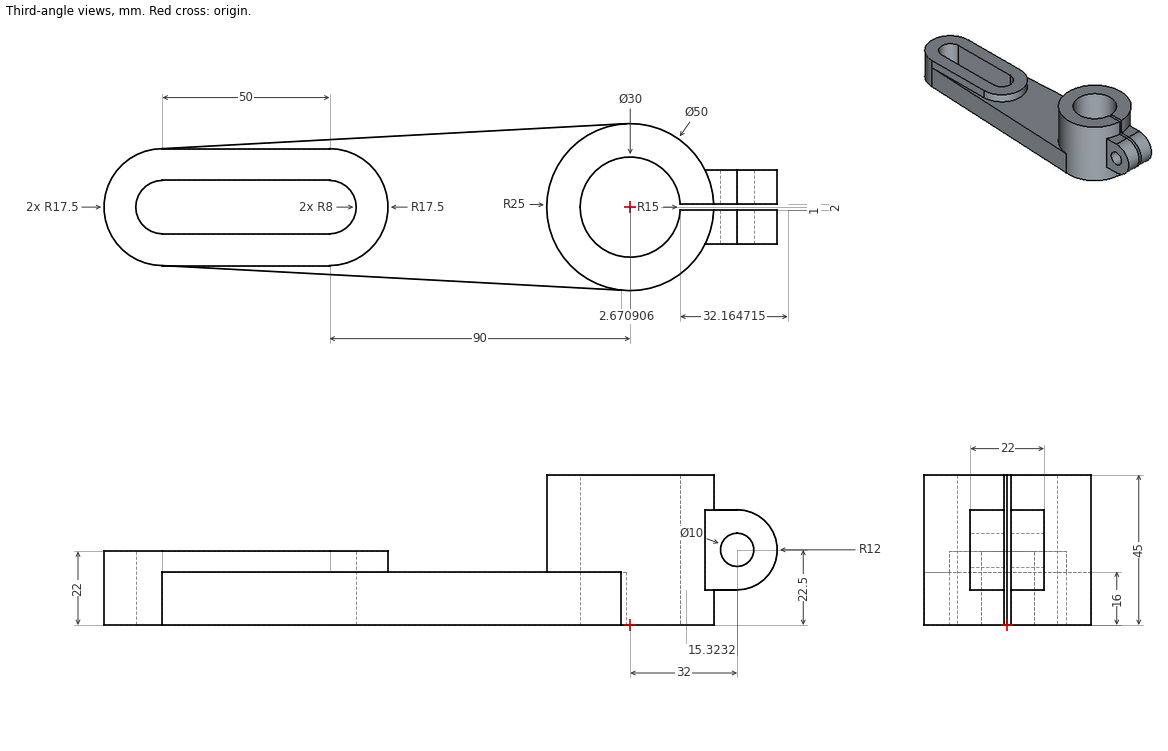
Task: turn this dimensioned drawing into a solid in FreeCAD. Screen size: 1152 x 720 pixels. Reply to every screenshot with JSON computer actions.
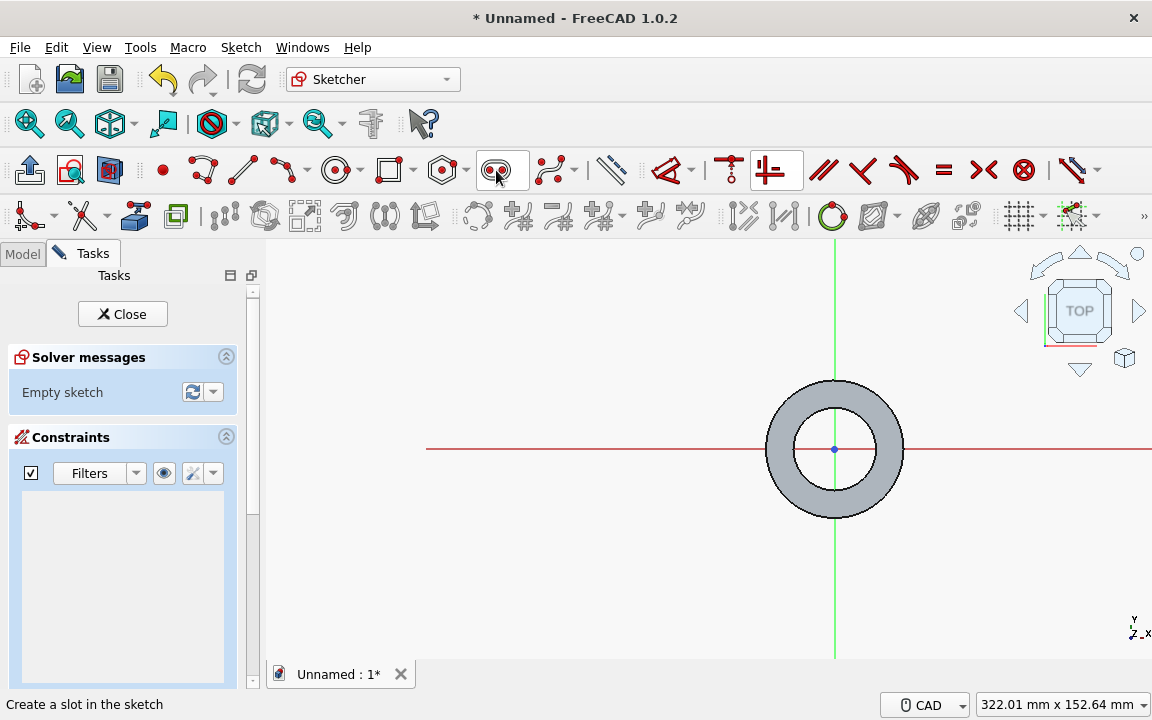
{"action": "left_click", "coordinate": [450, 449]}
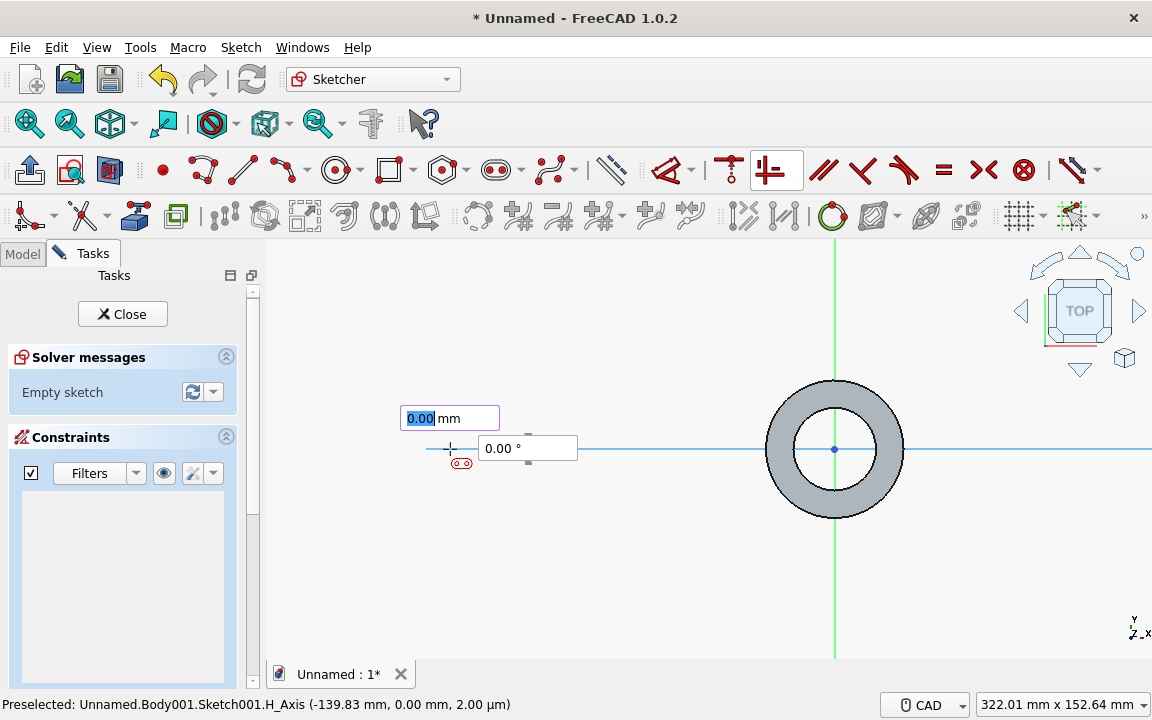
{"action": "left_click", "coordinate": [587, 440]}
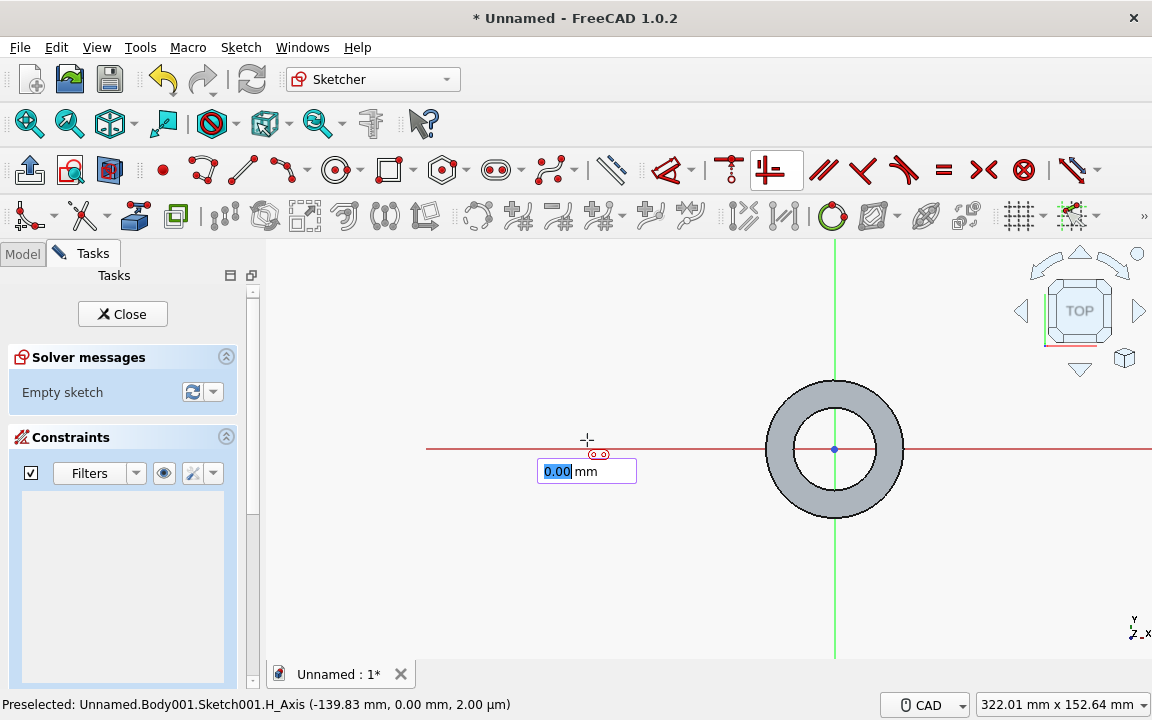
{"action": "left_click", "coordinate": [518, 401]}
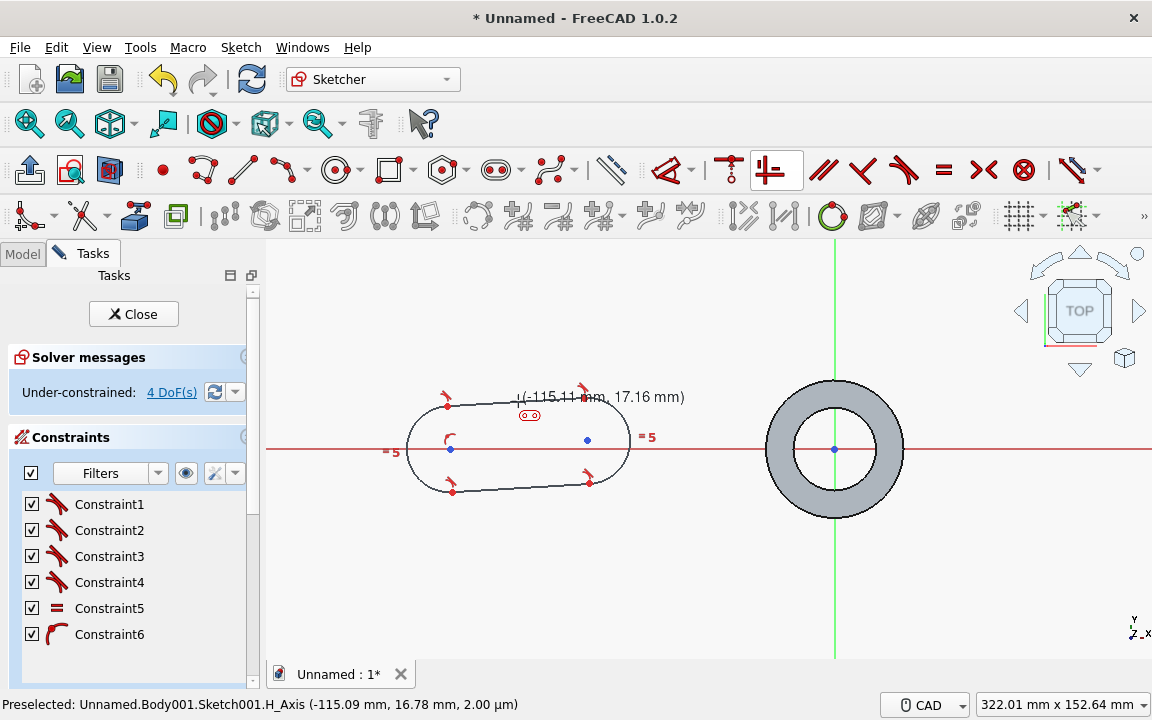
{"action": "left_click", "coordinate": [450, 449]}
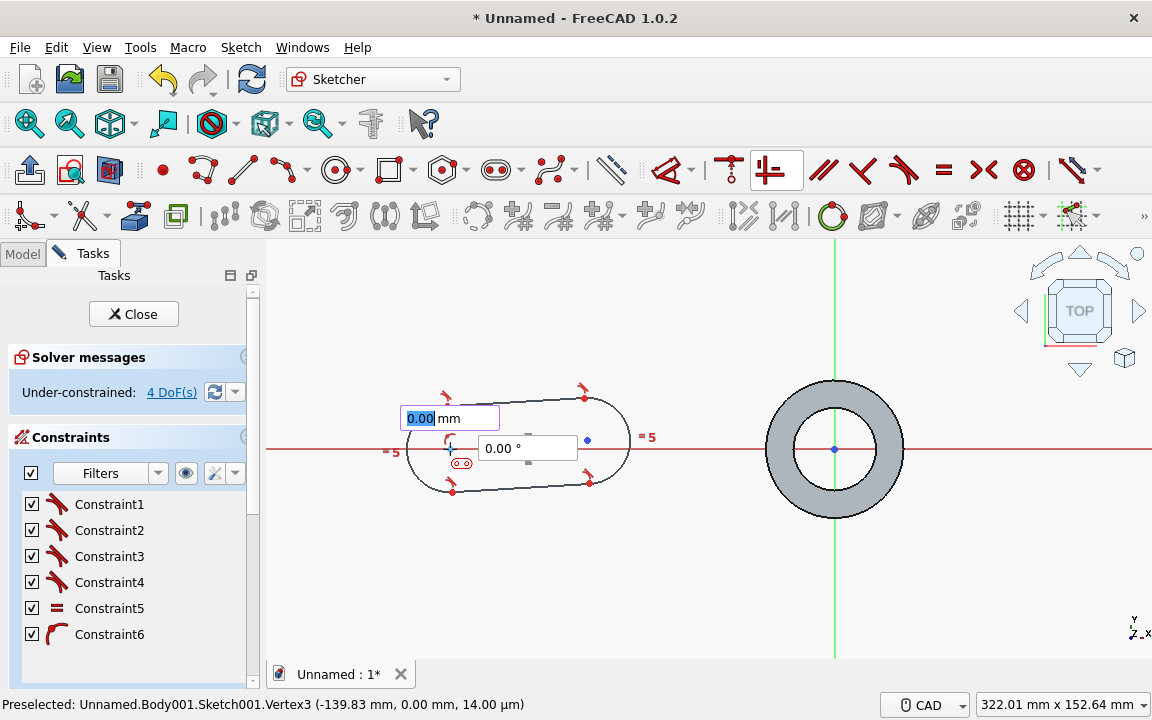
{"action": "left_click", "coordinate": [587, 441]}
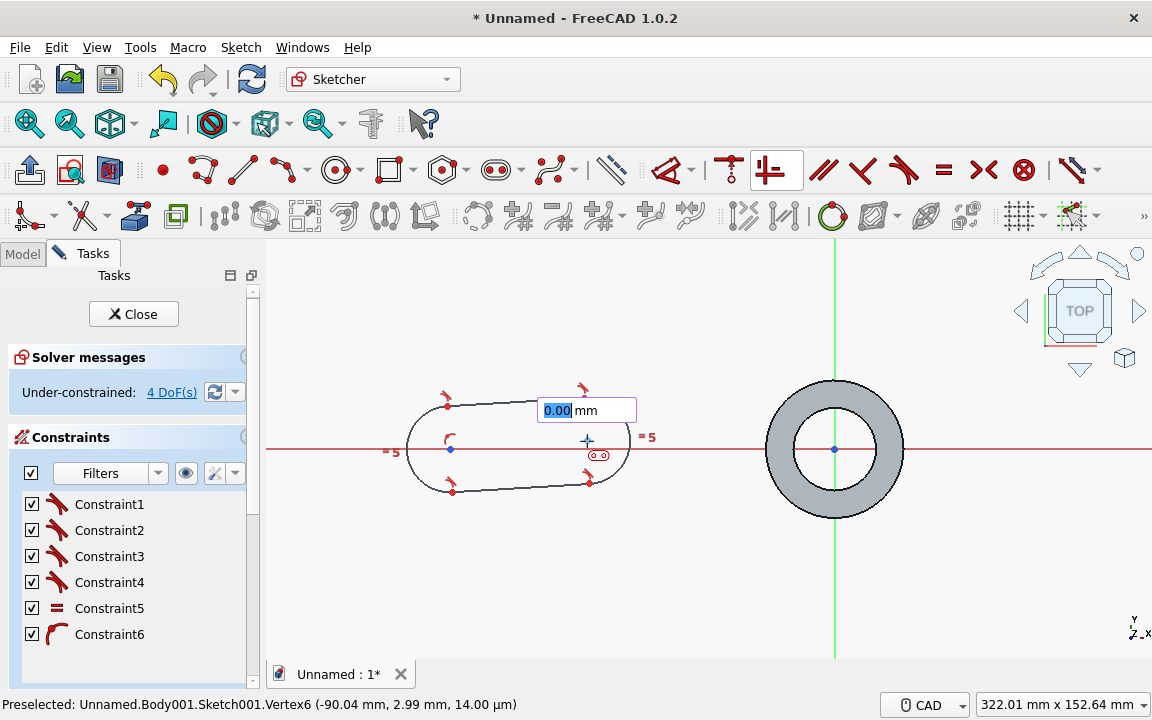
{"action": "left_click", "coordinate": [518, 427]}
{"action": "key", "text": "Escape"}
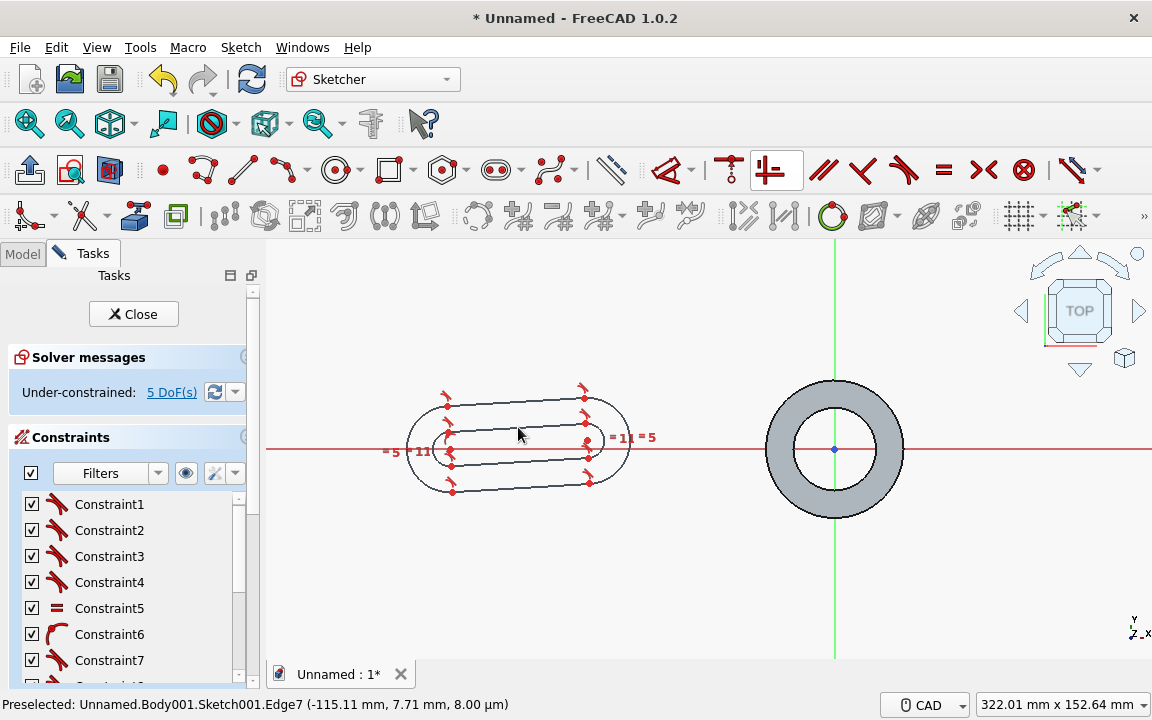
{"action": "left_click", "coordinate": [489, 404]}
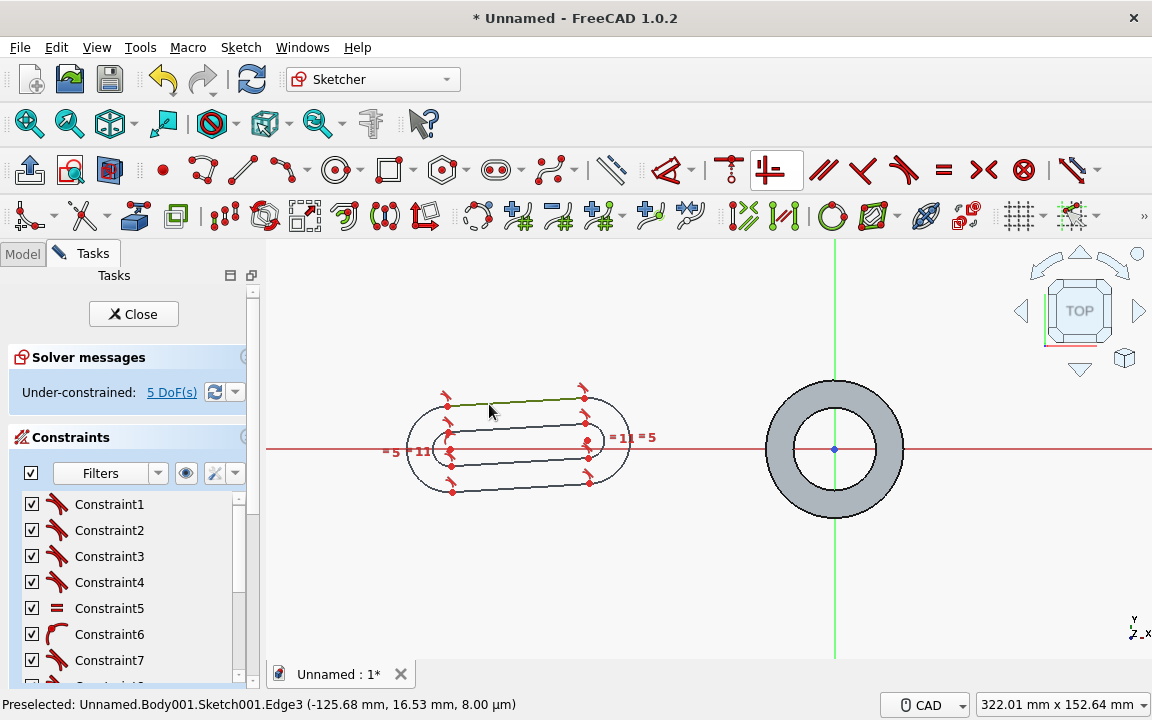
{"action": "key", "text": "h"}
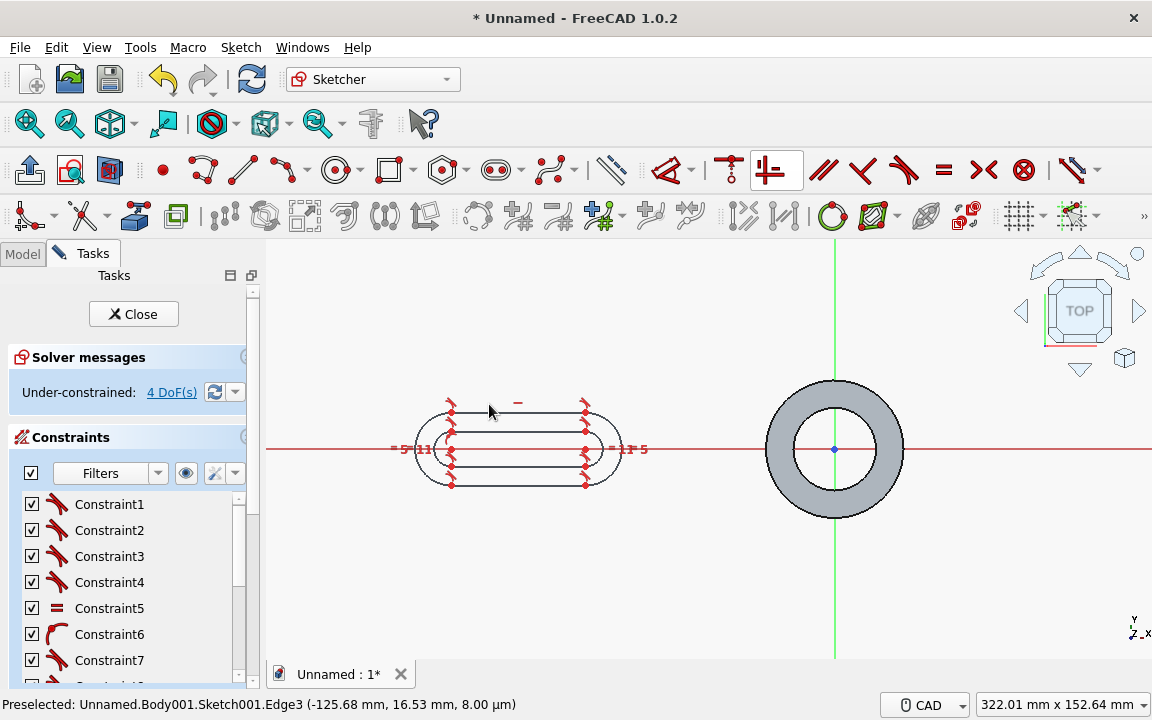
{"action": "left_click", "coordinate": [666, 170]}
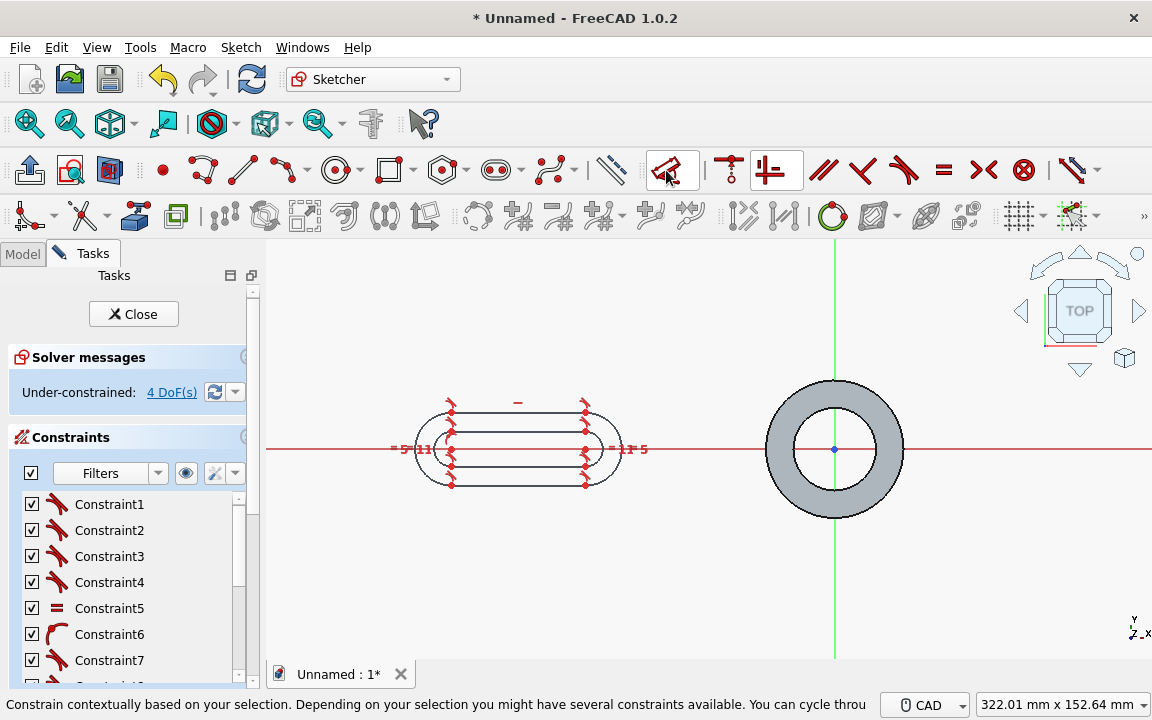
{"action": "left_click", "coordinate": [422, 428]}
{"action": "left_click", "coordinate": [396, 409]}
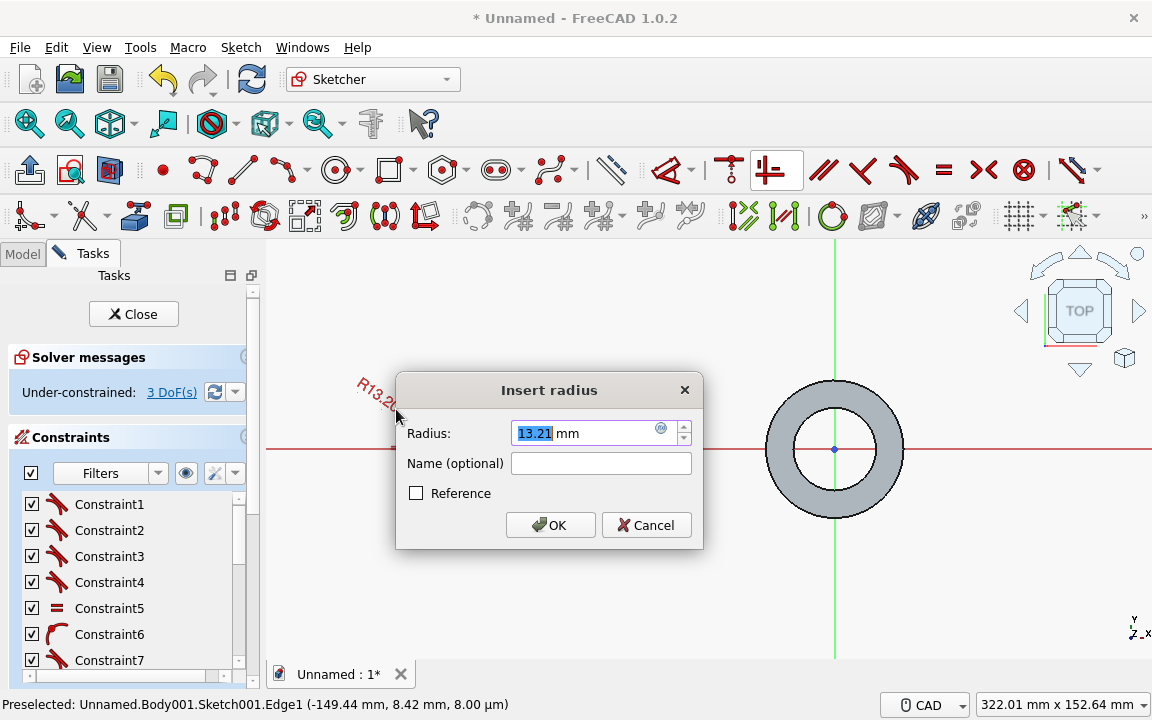
{"action": "type", "text": "17.5"}
{"action": "key", "text": "Return"}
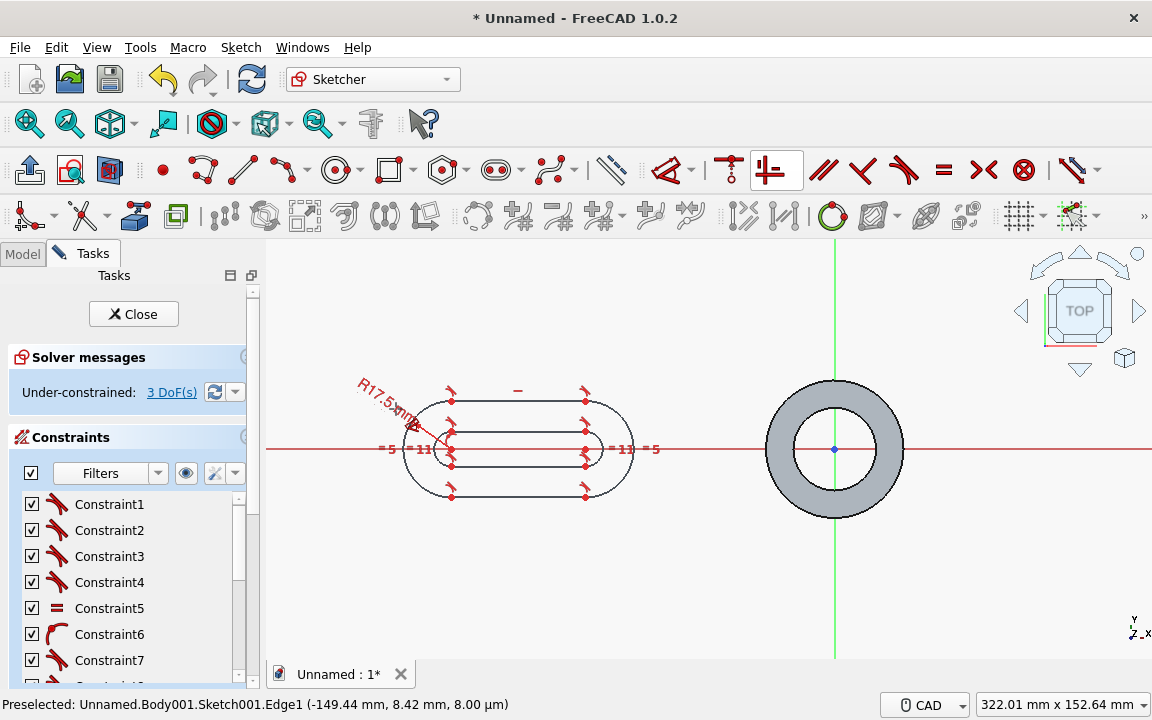
{"action": "scroll", "coordinate": [438, 439], "scroll_direction": "up", "scroll_amount": 3}